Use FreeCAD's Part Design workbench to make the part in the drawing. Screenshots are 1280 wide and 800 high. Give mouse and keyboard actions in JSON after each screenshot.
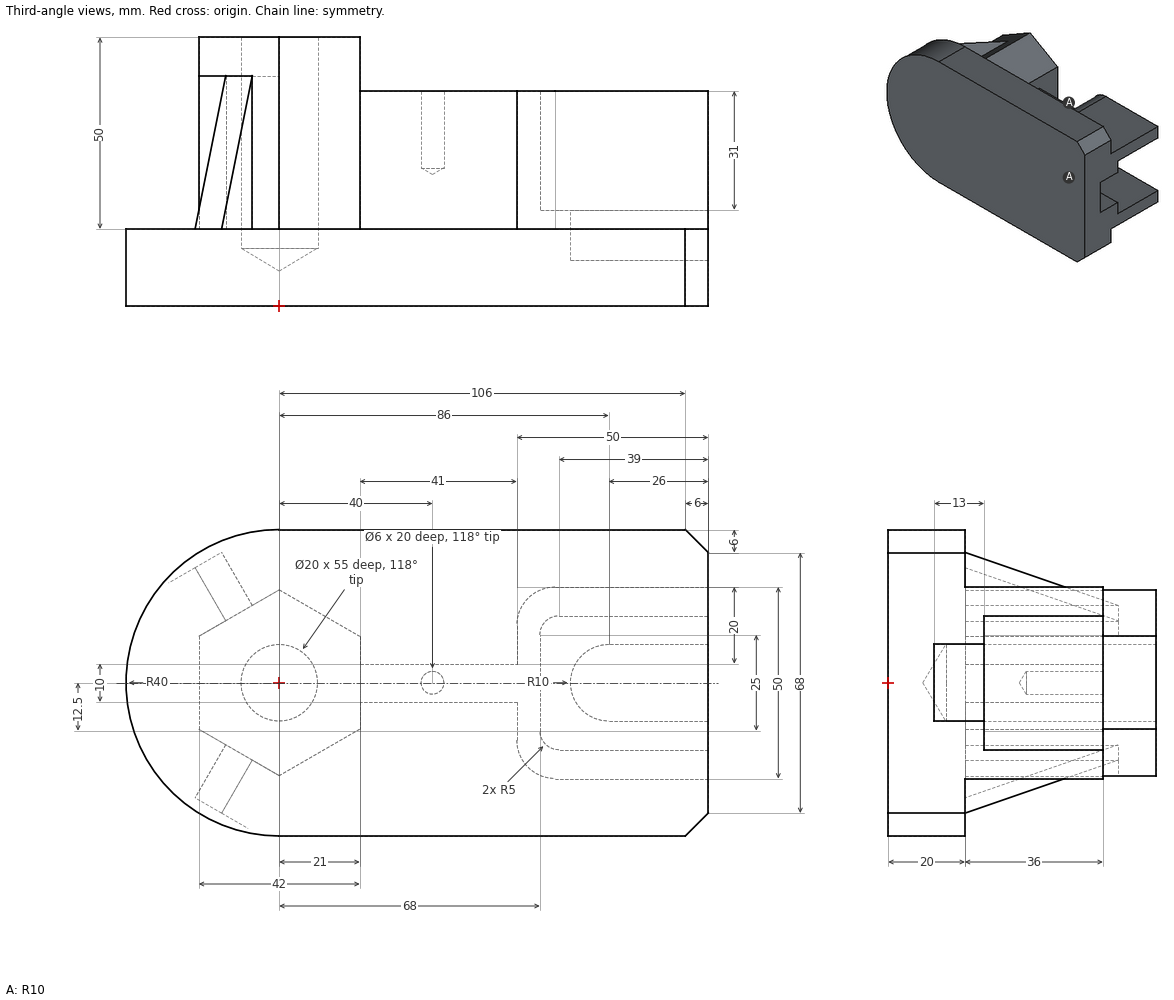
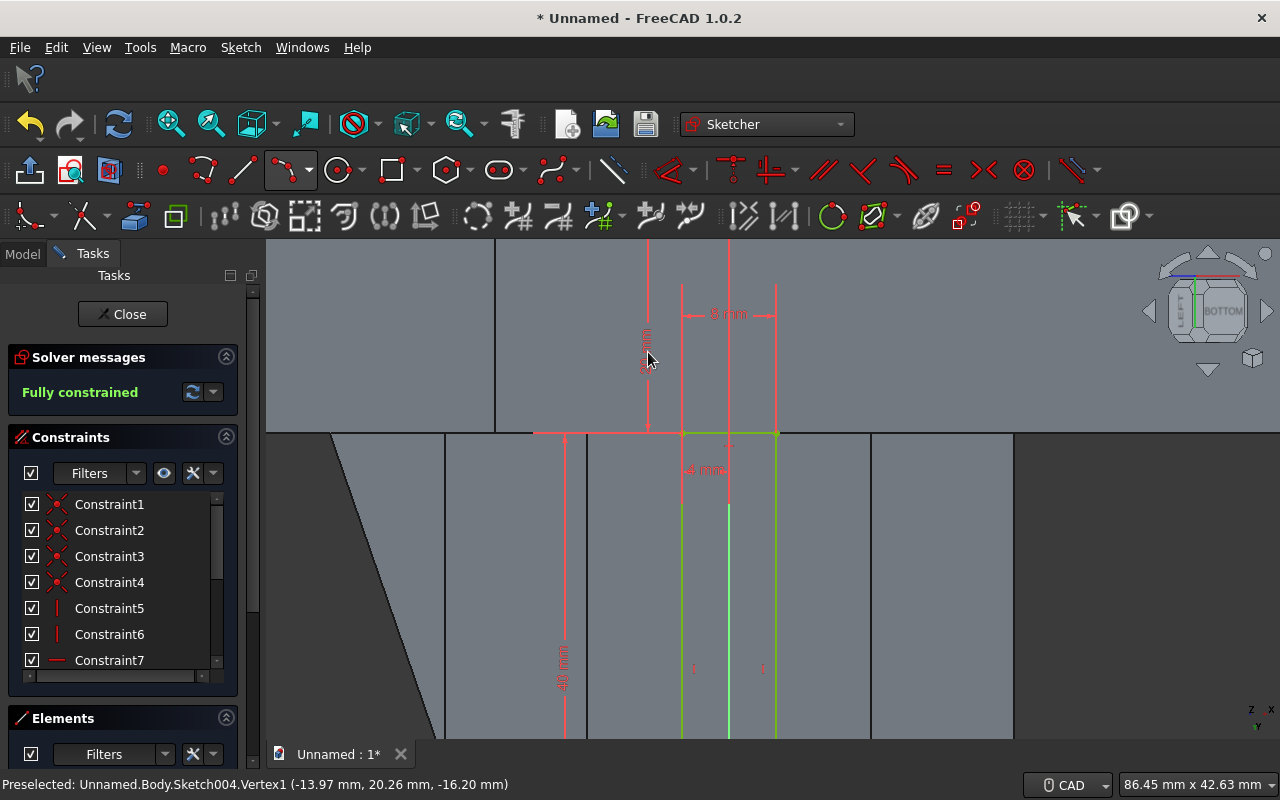
{"action": "left_click", "coordinate": [123, 314]}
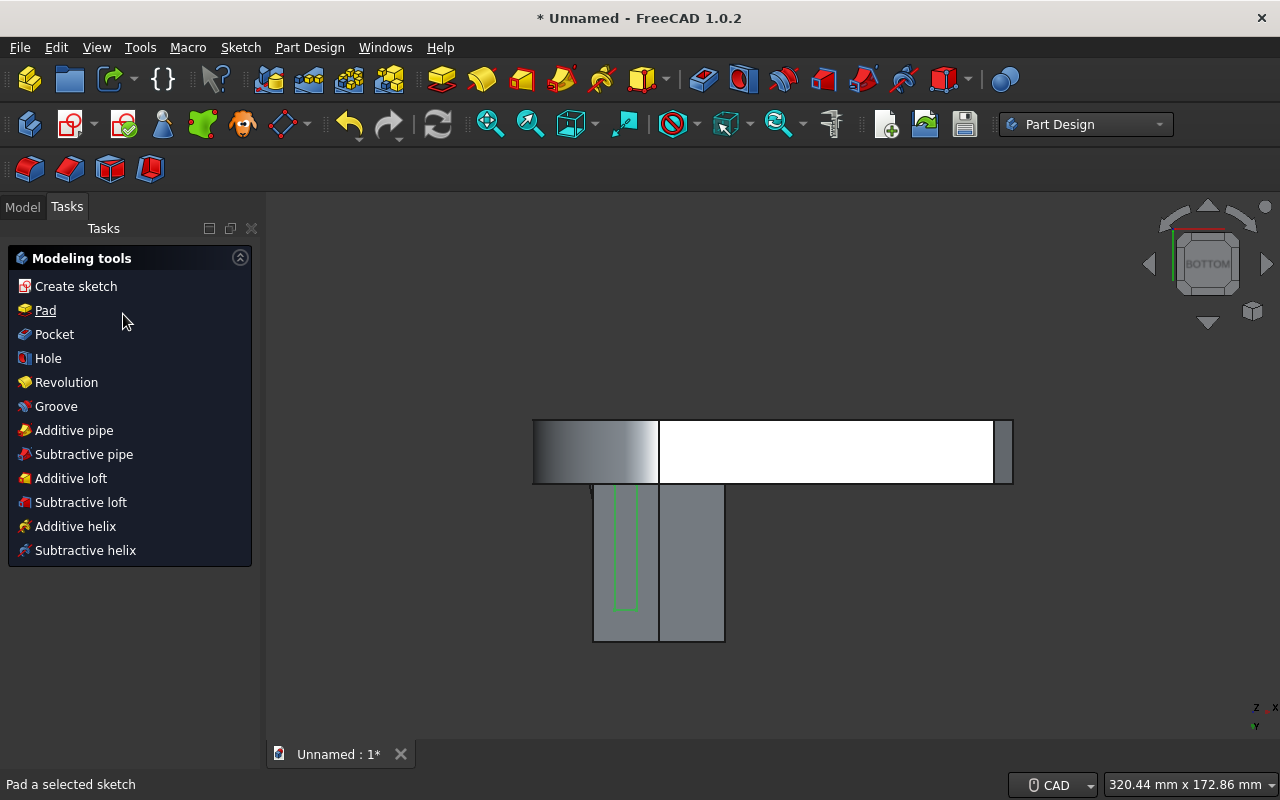
{"action": "left_click", "coordinate": [442, 80]}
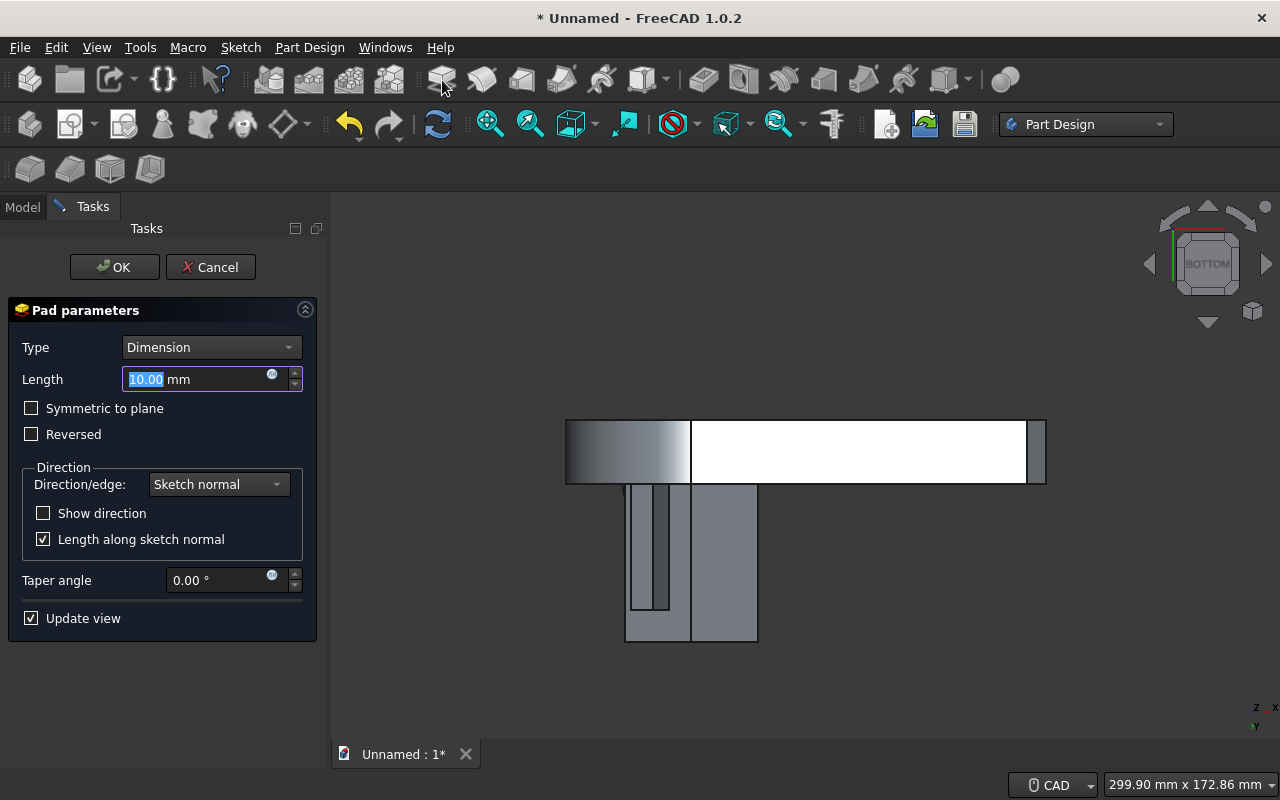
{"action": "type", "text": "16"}
{"action": "key", "text": "Tab"}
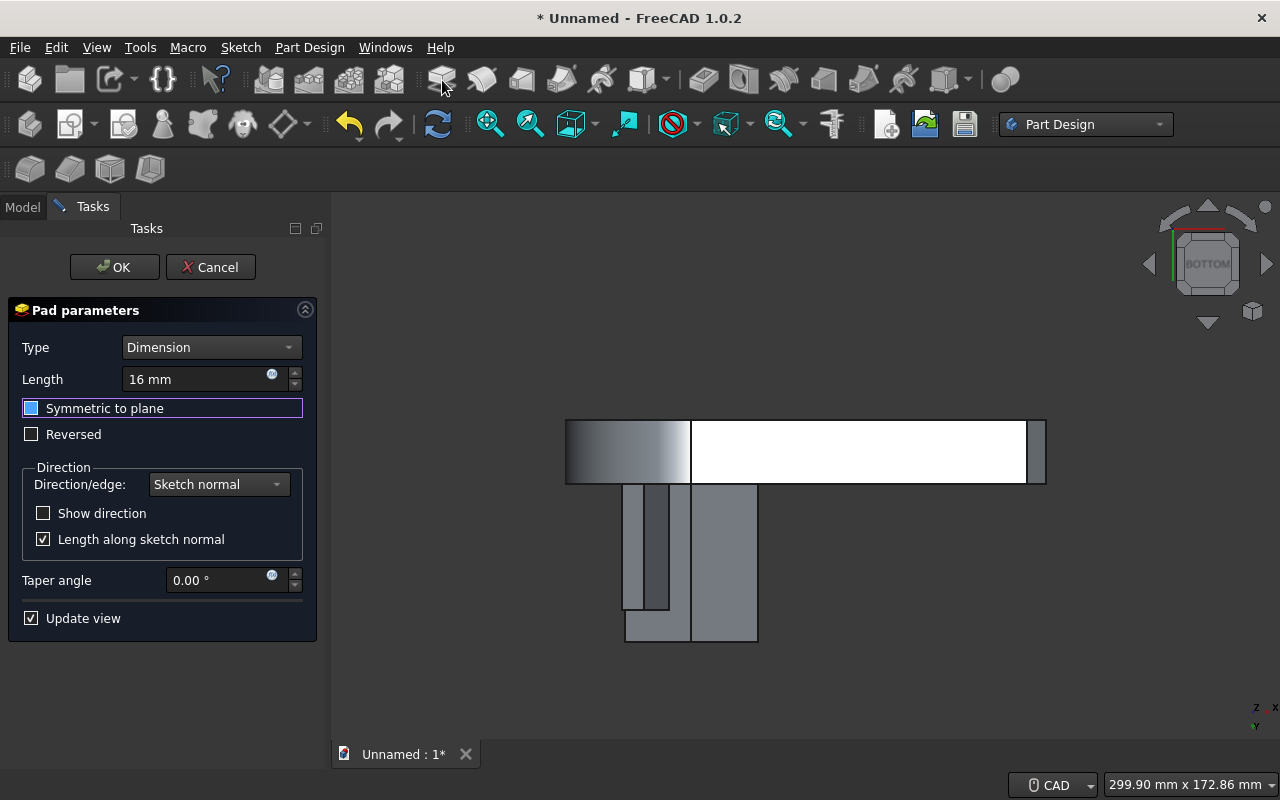
{"action": "left_click", "coordinate": [115, 267]}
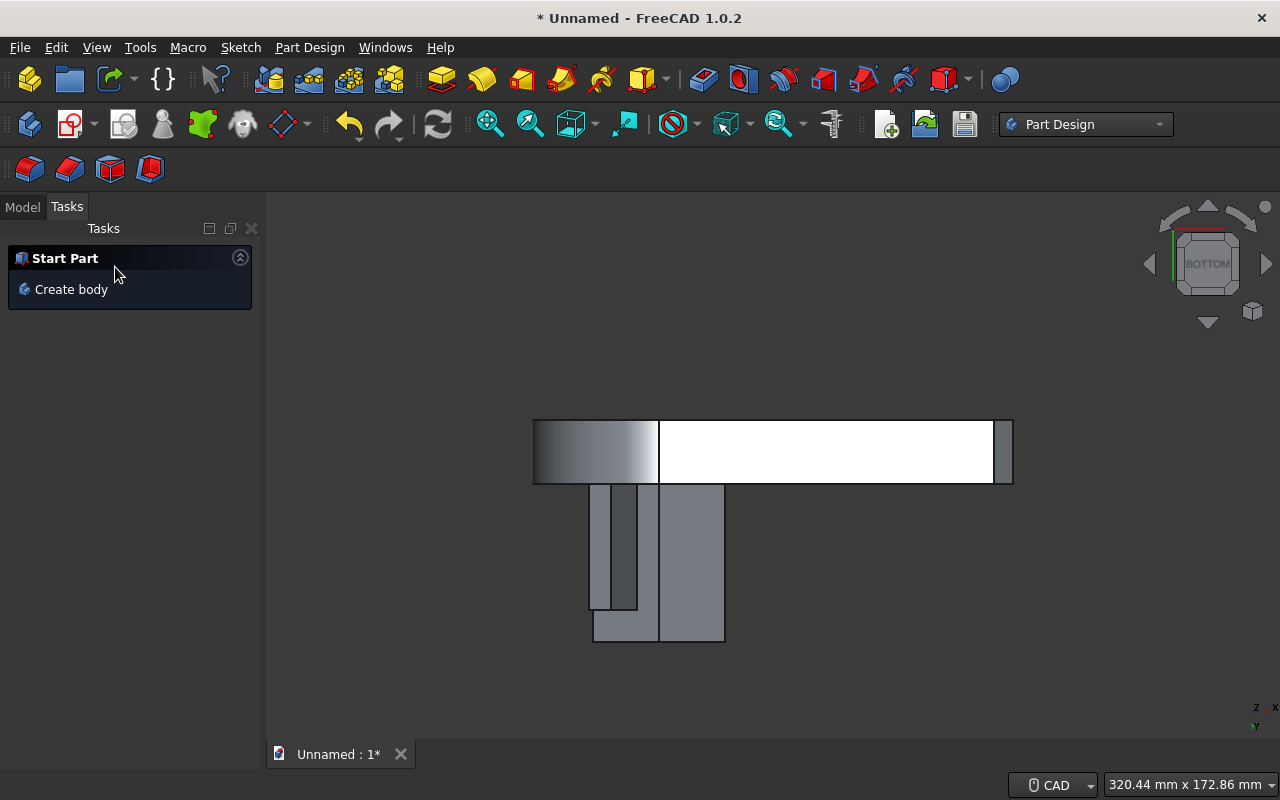
{"action": "key", "text": "6"}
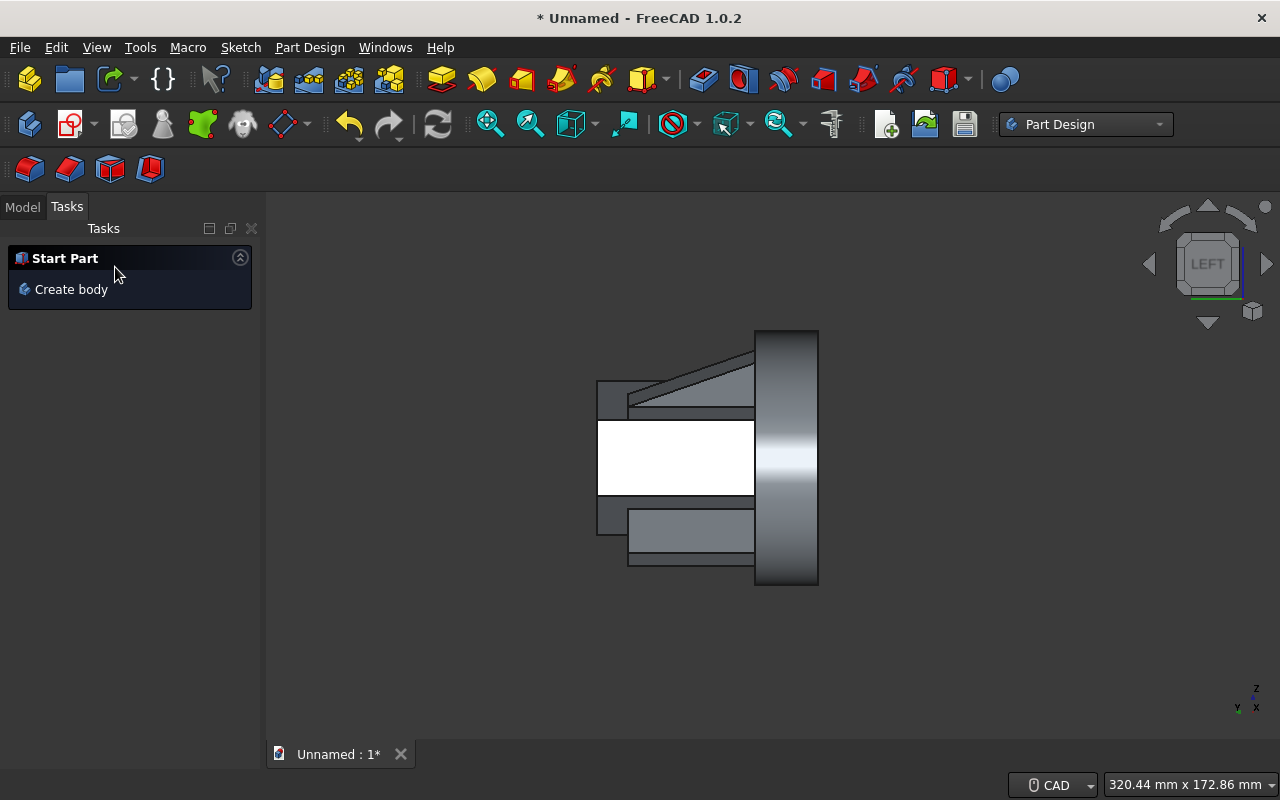
{"action": "left_click", "coordinate": [655, 530]}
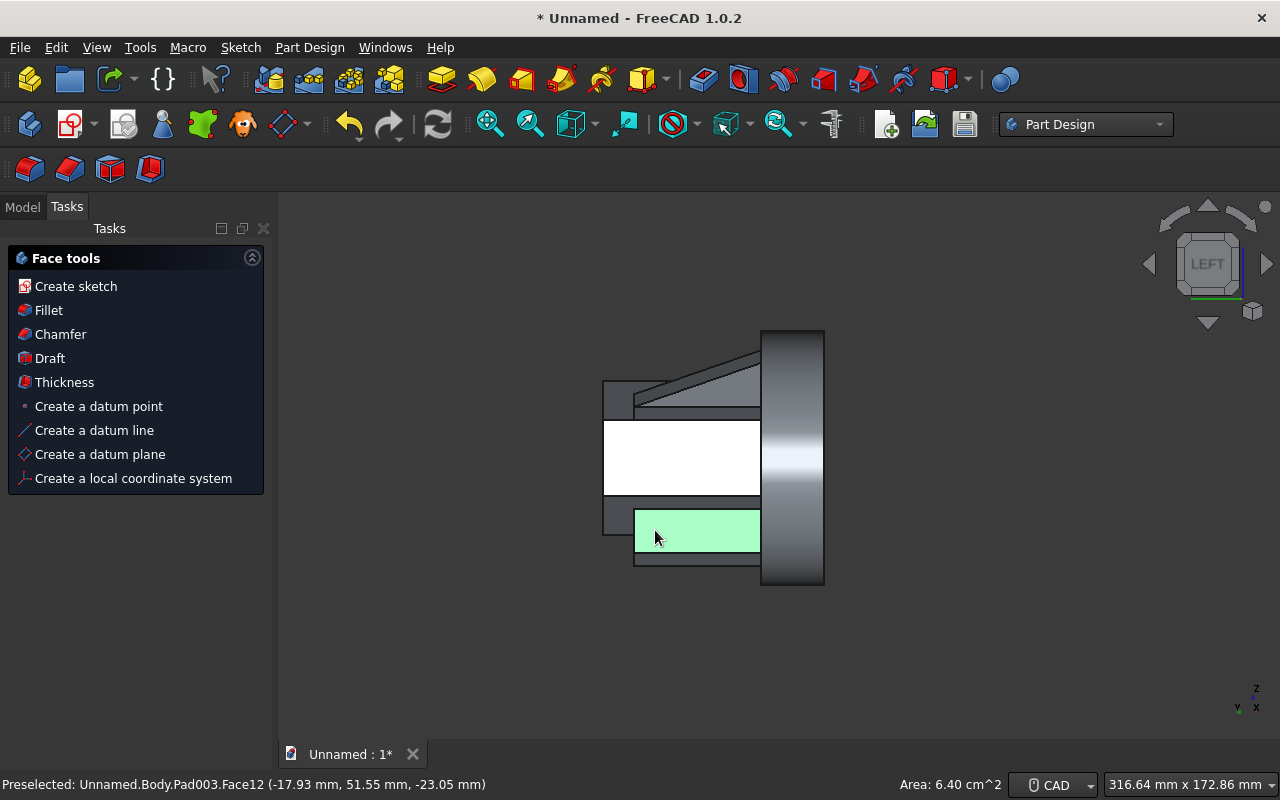
{"action": "left_click", "coordinate": [70, 124]}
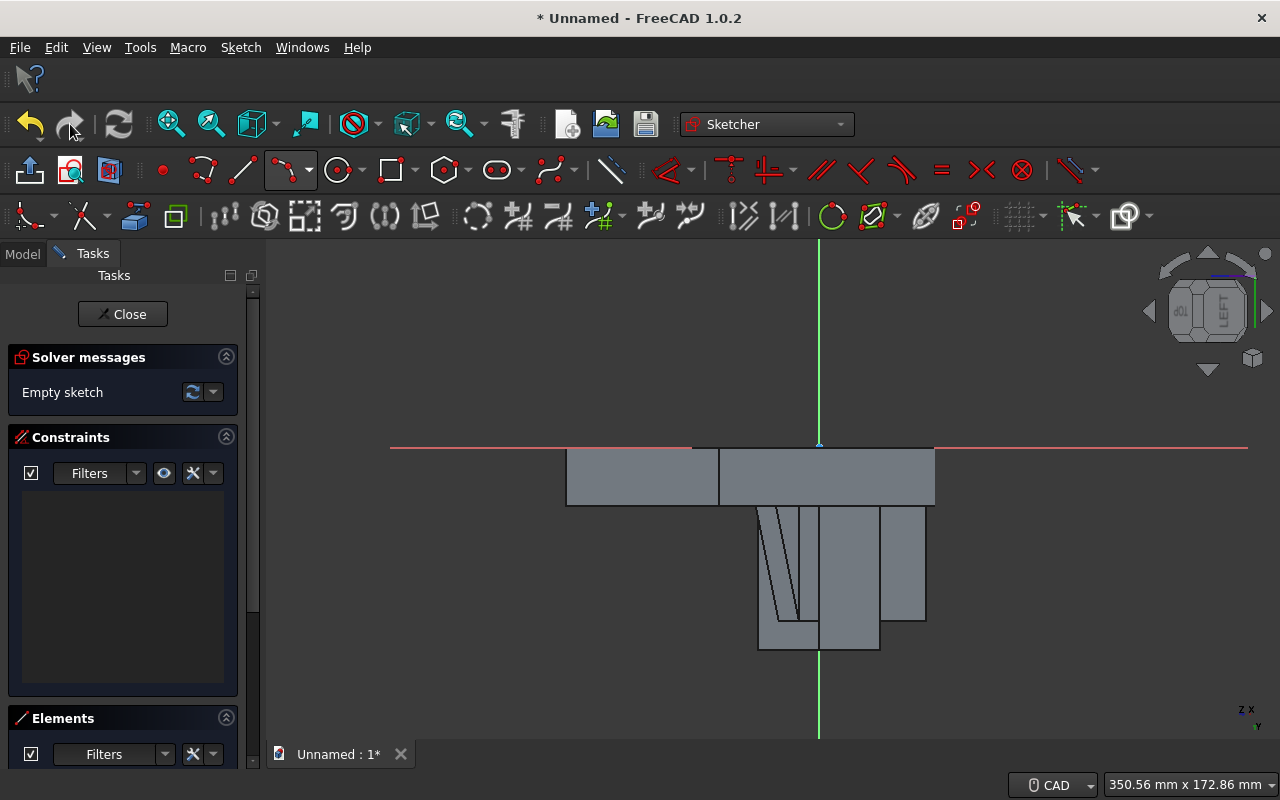
{"action": "left_click", "coordinate": [110, 170]}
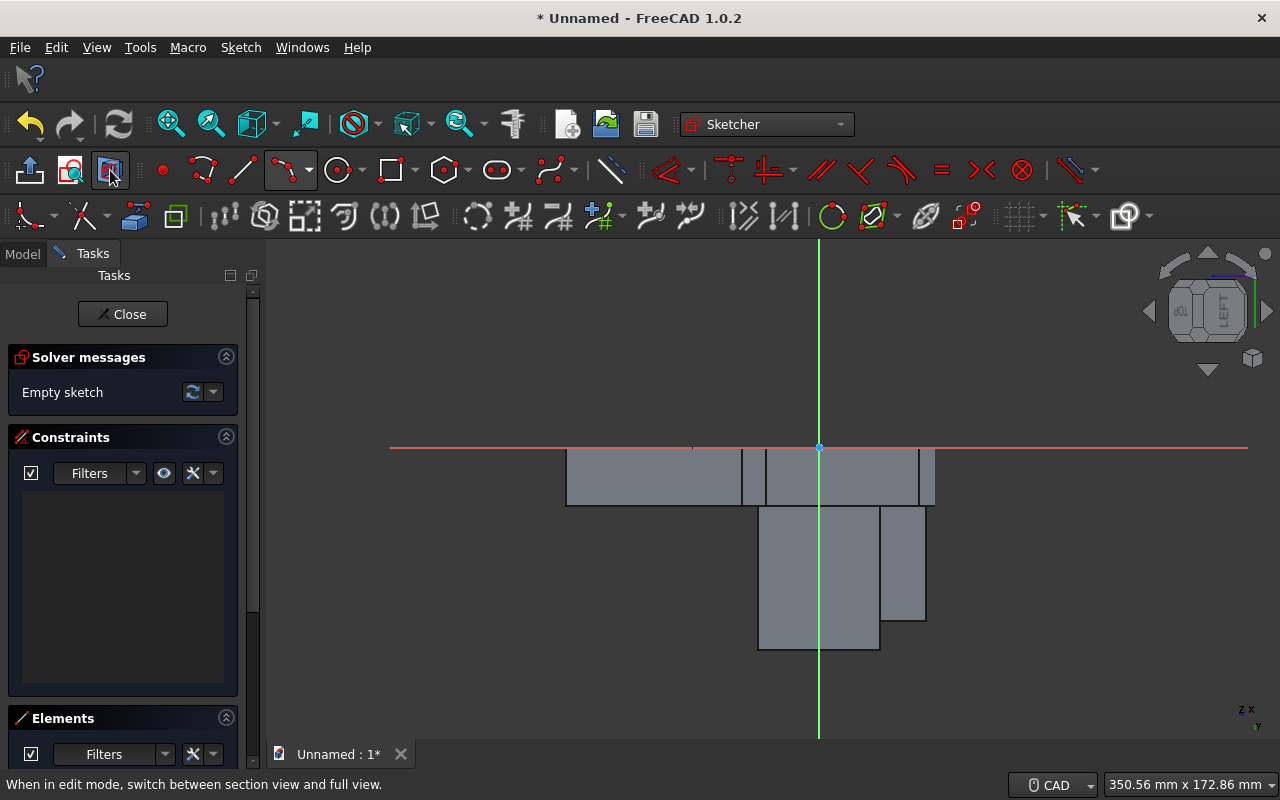
{"action": "scroll", "coordinate": [1077, 590], "scroll_direction": "up", "scroll_amount": 3}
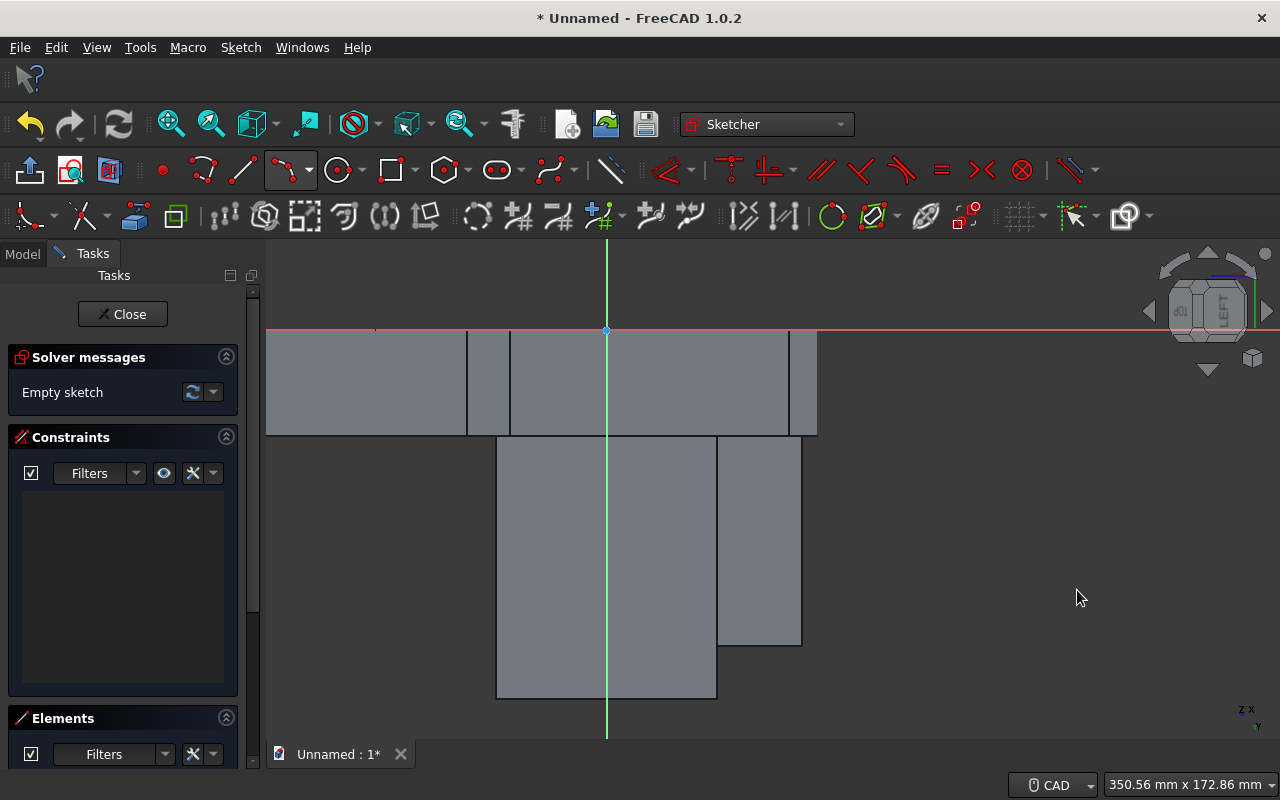
{"action": "left_click", "coordinate": [204, 170]}